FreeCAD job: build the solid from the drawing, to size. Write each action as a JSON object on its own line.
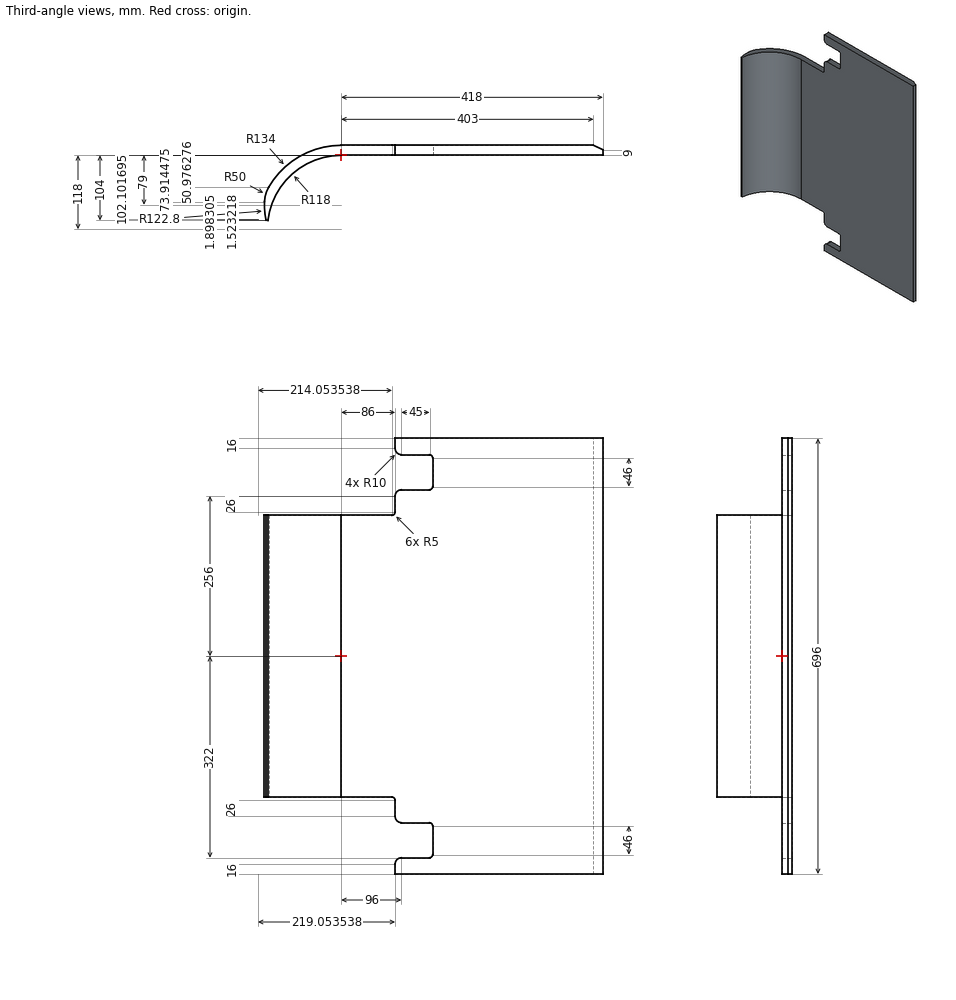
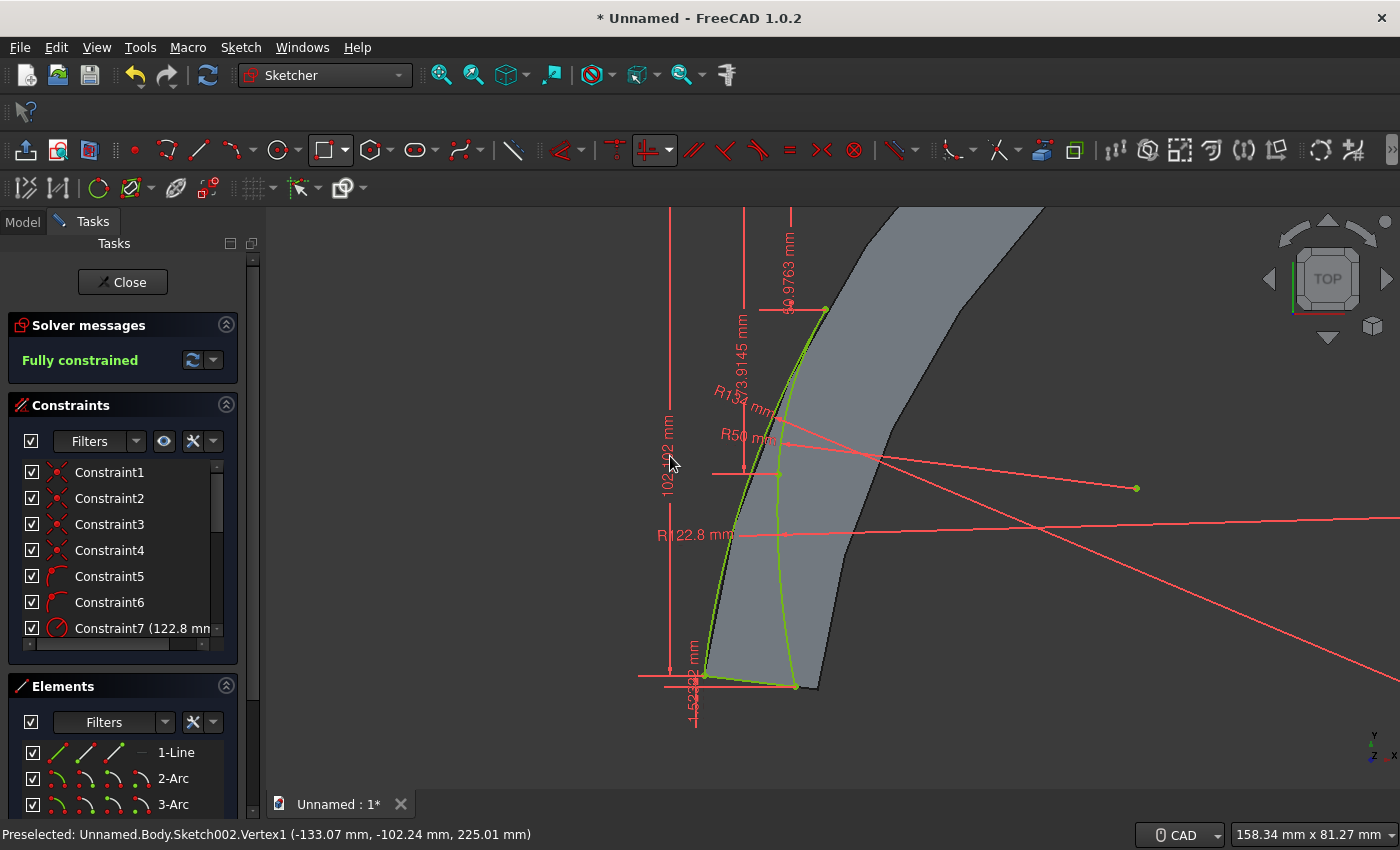
{"action": "left_click", "coordinate": [123, 282]}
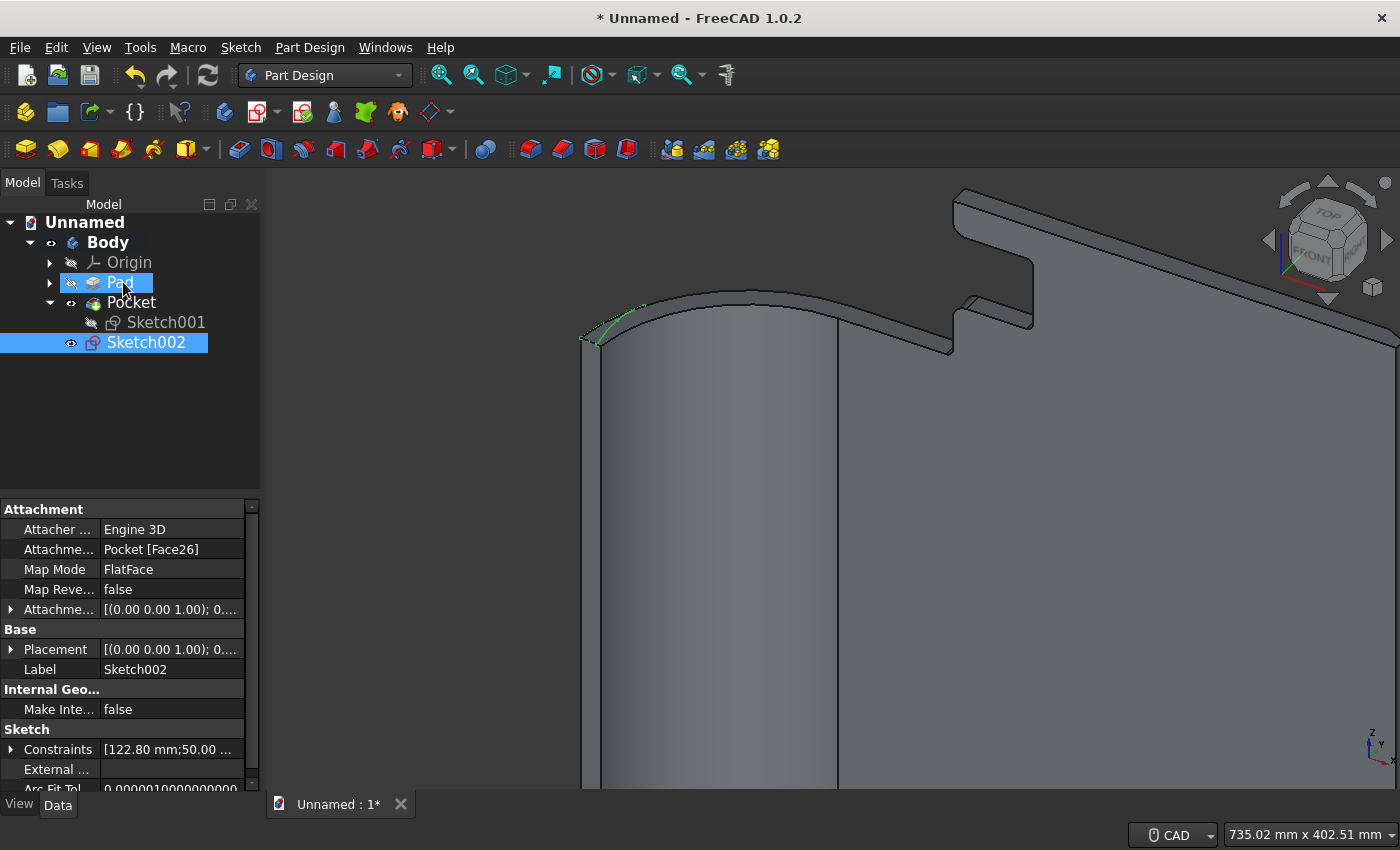
{"action": "left_click", "coordinate": [240, 150]}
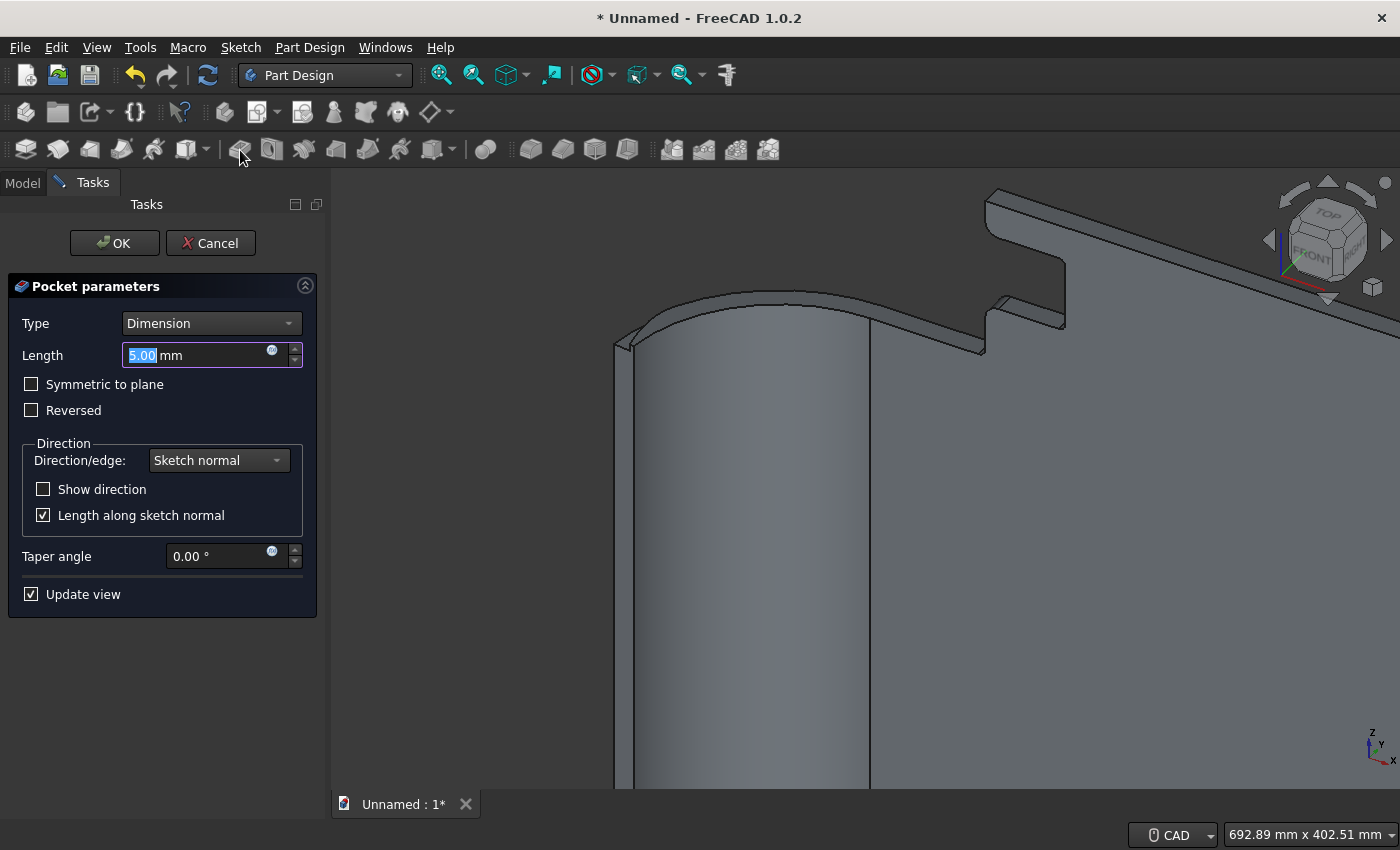
{"action": "left_click", "coordinate": [212, 324]}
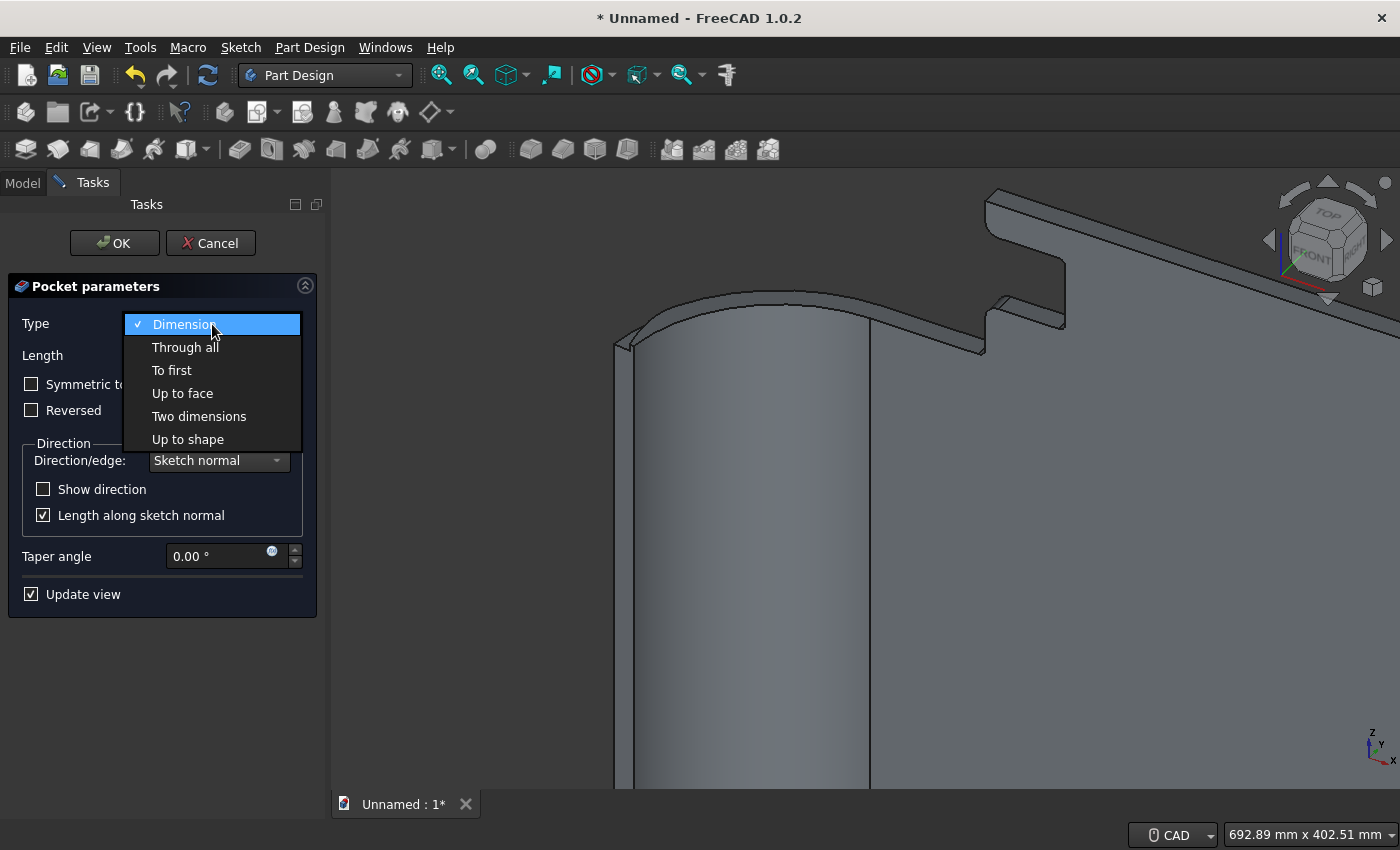
{"action": "left_click", "coordinate": [212, 348]}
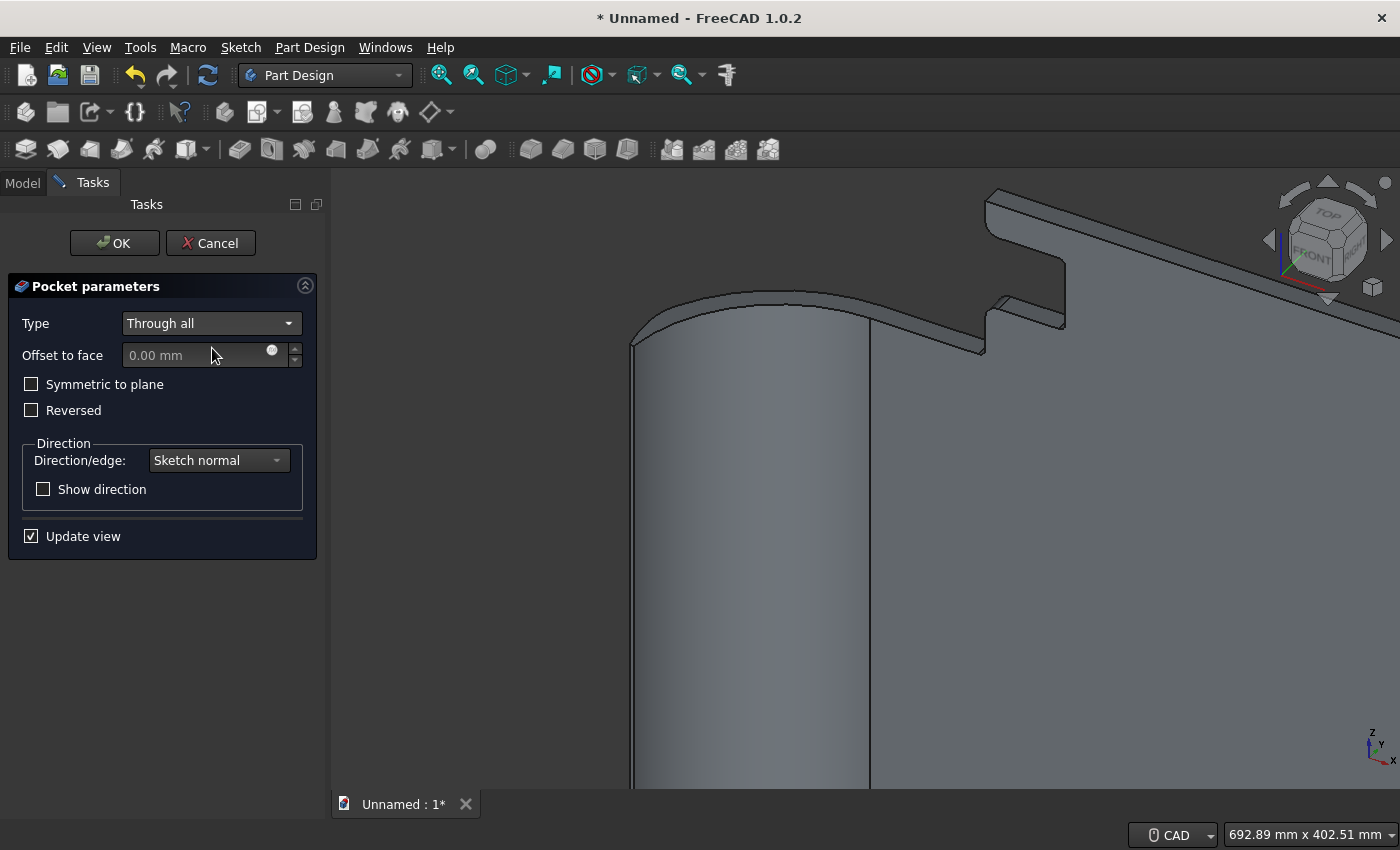
{"action": "left_click", "coordinate": [115, 243]}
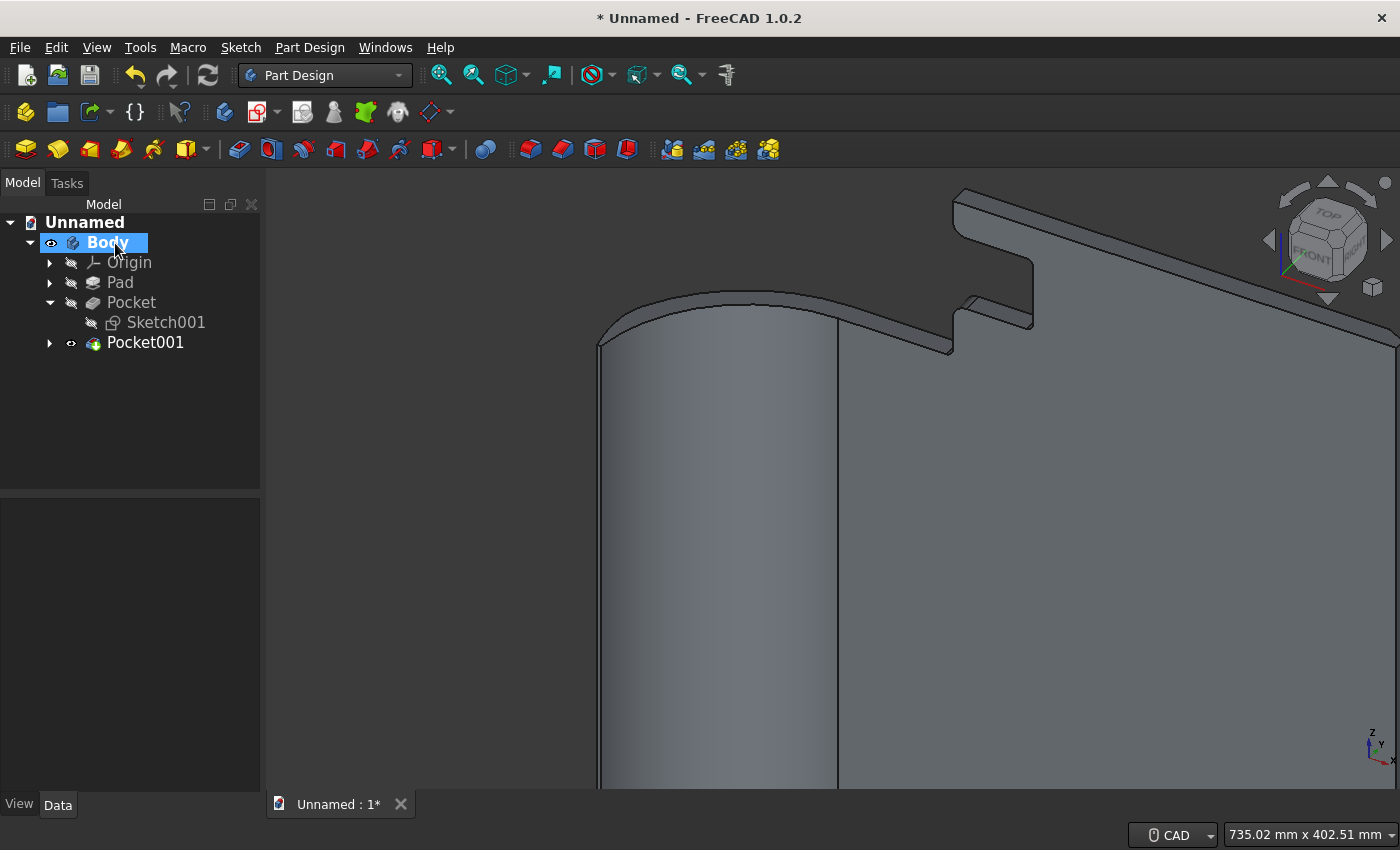
{"action": "key", "text": "0"}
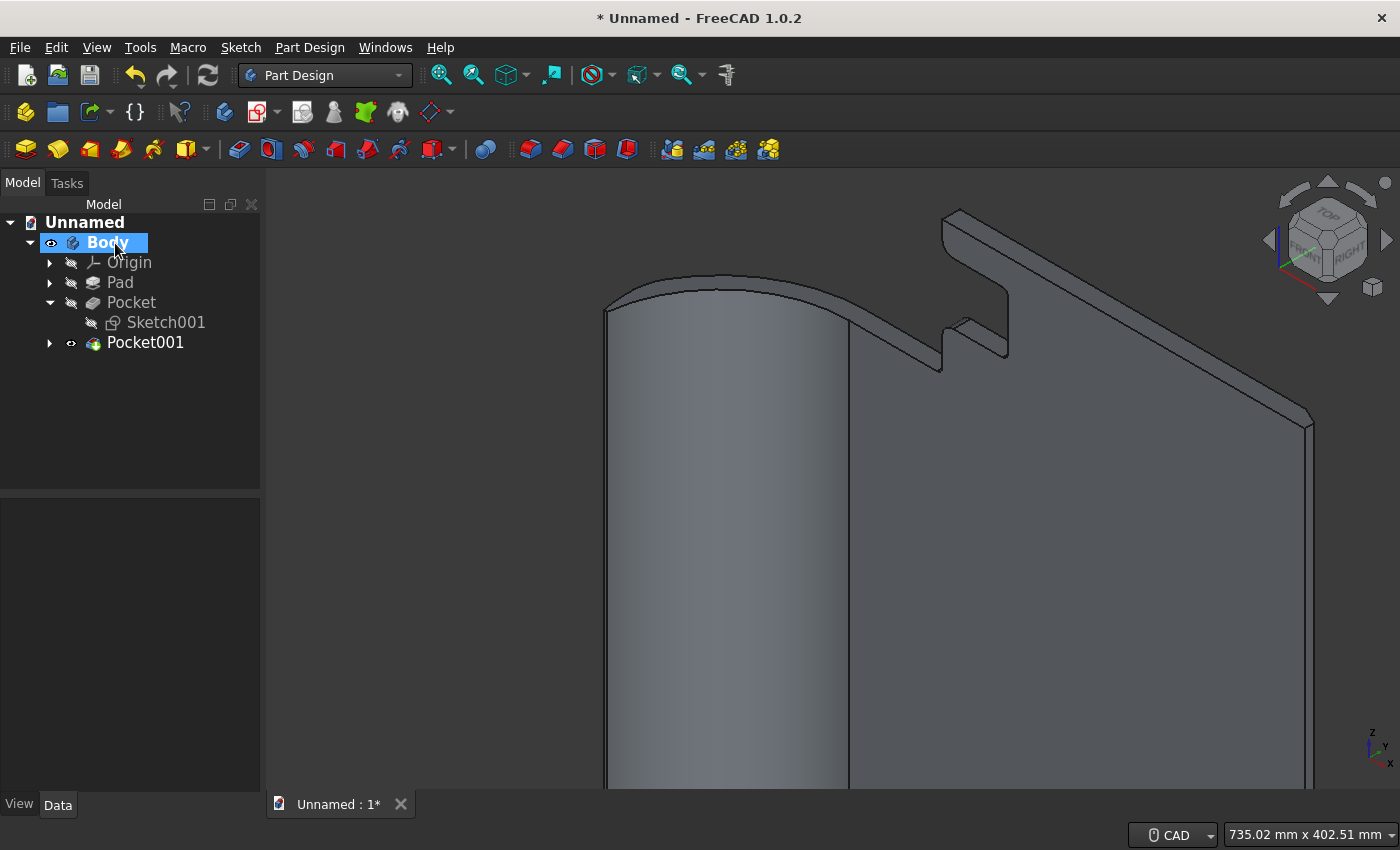
{"action": "left_click", "coordinate": [442, 76]}